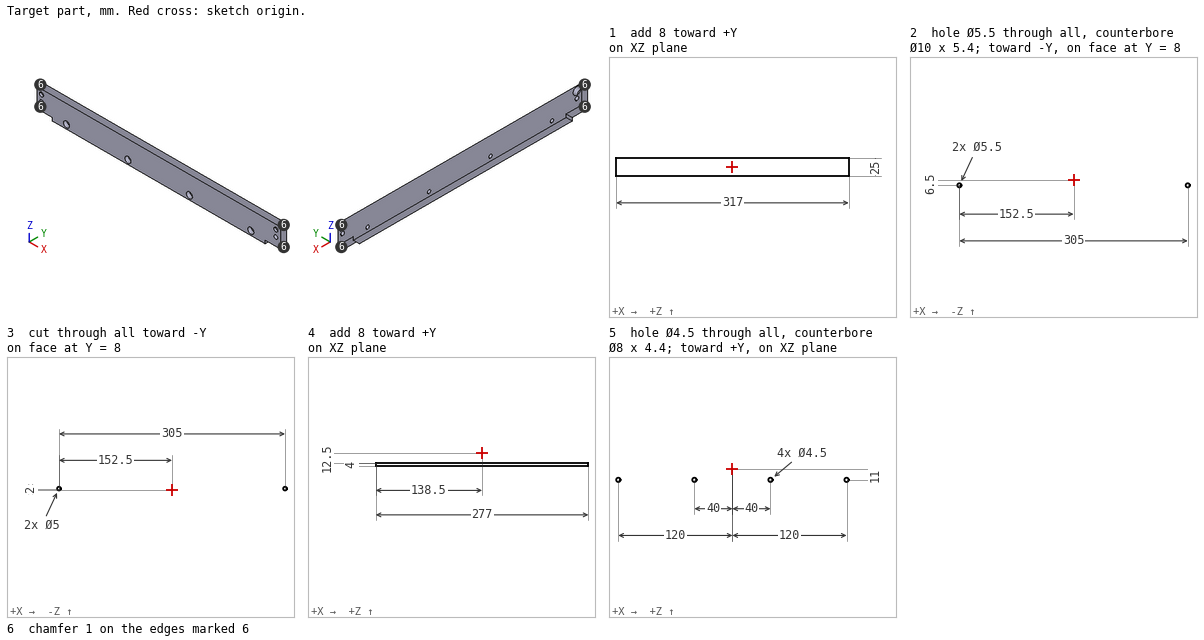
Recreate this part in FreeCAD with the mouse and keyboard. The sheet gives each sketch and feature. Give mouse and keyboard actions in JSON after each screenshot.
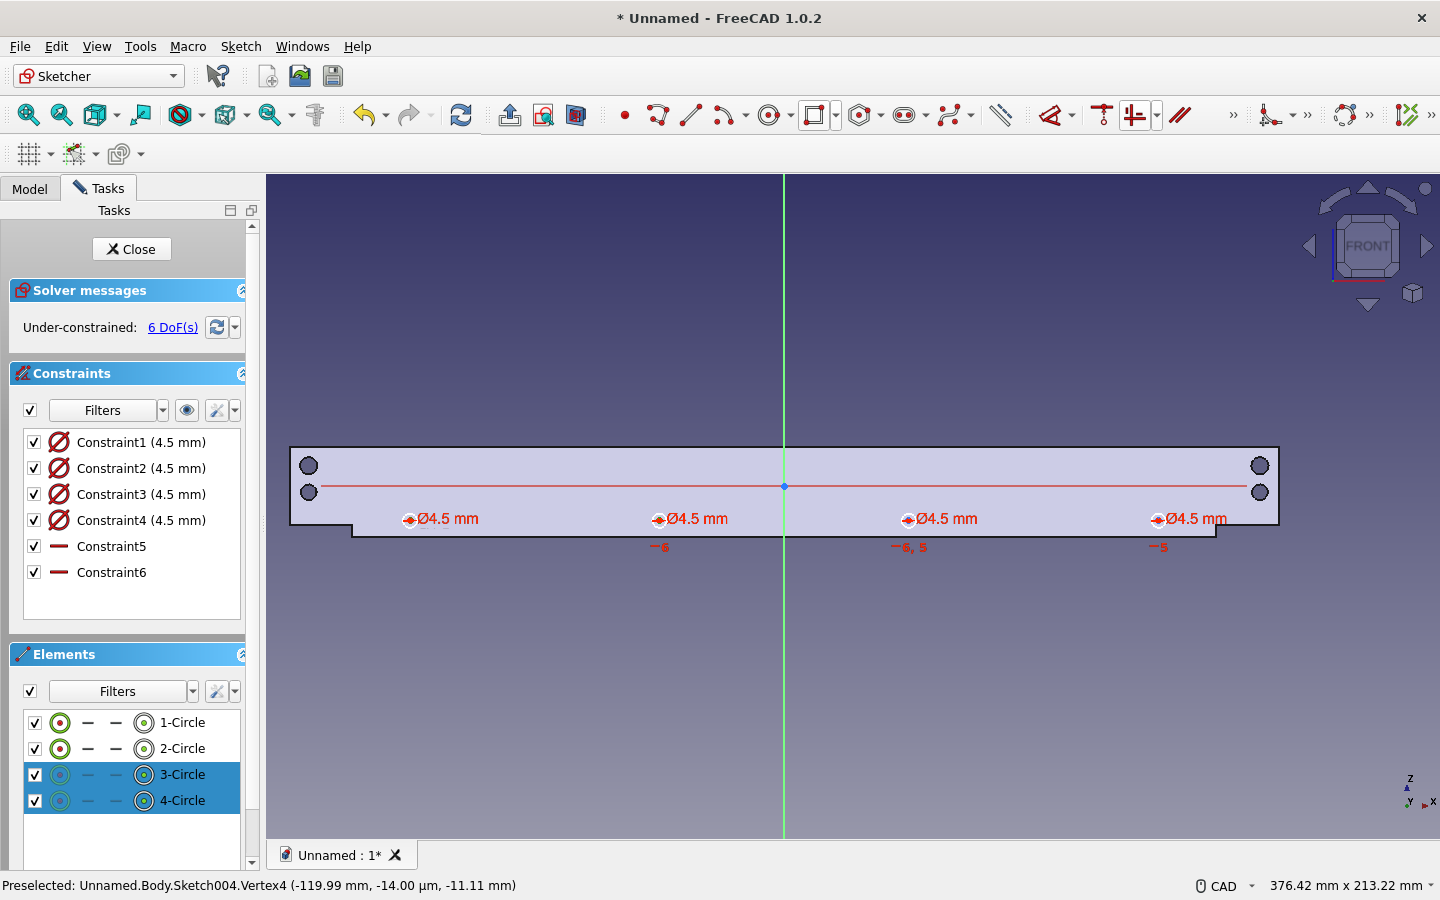
{"action": "left_click", "coordinate": [1156, 116]}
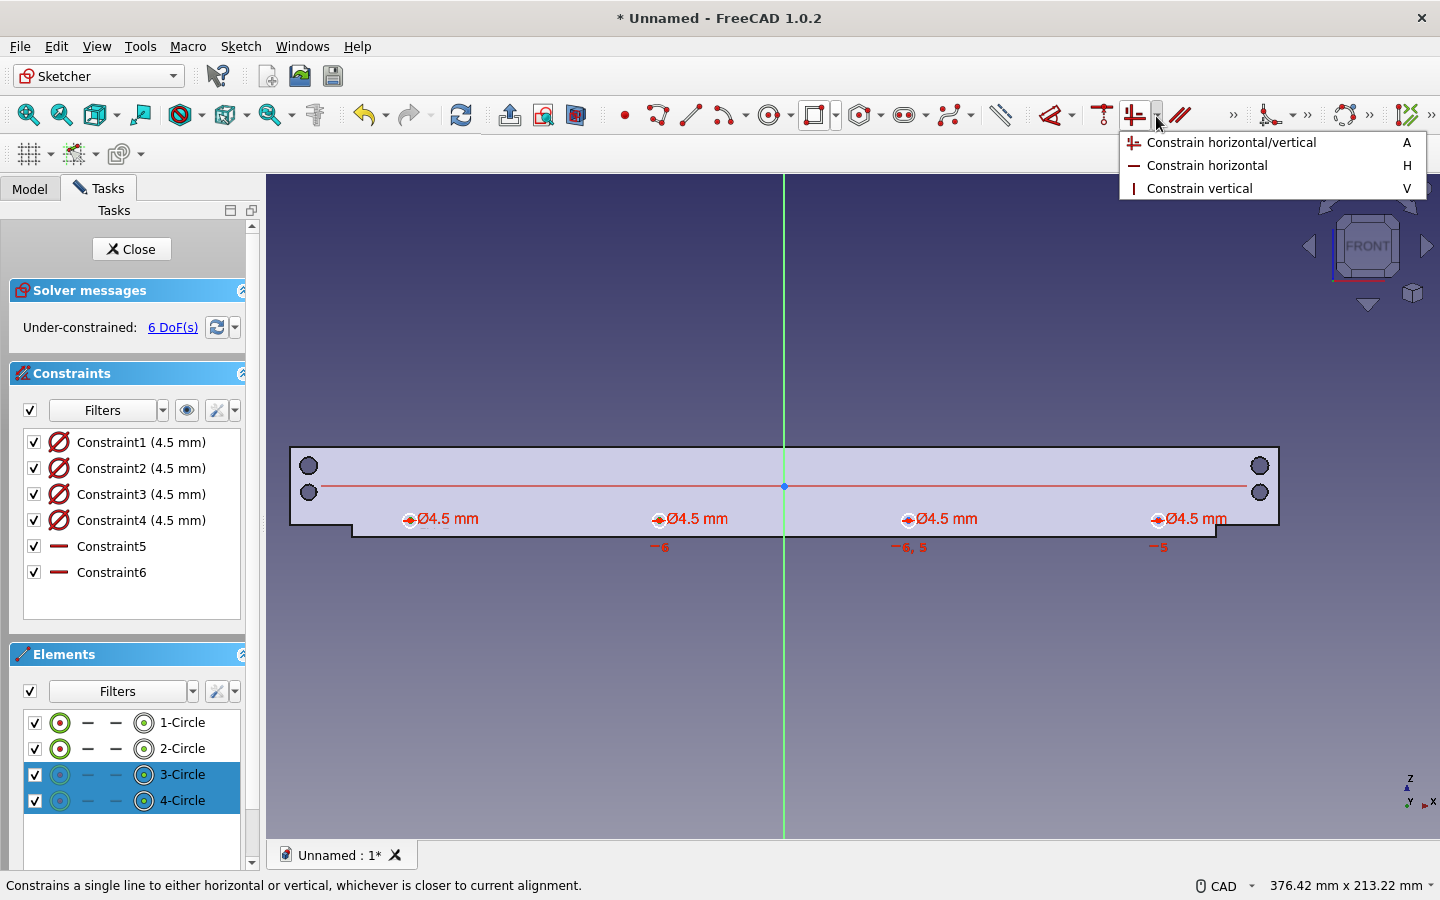
{"action": "left_click", "coordinate": [1273, 166]}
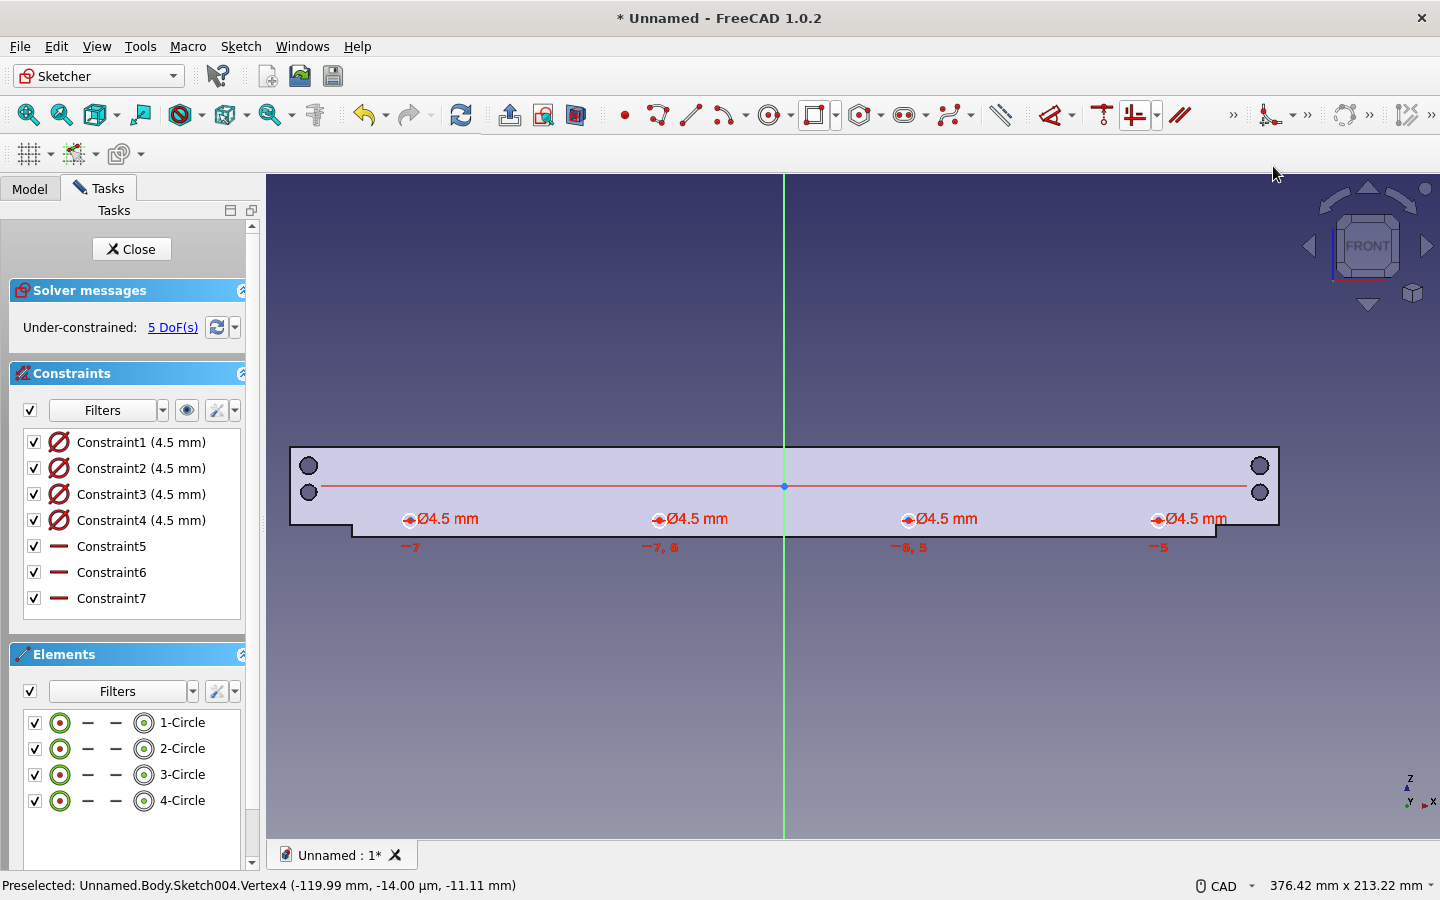
{"action": "left_click", "coordinate": [1050, 116]}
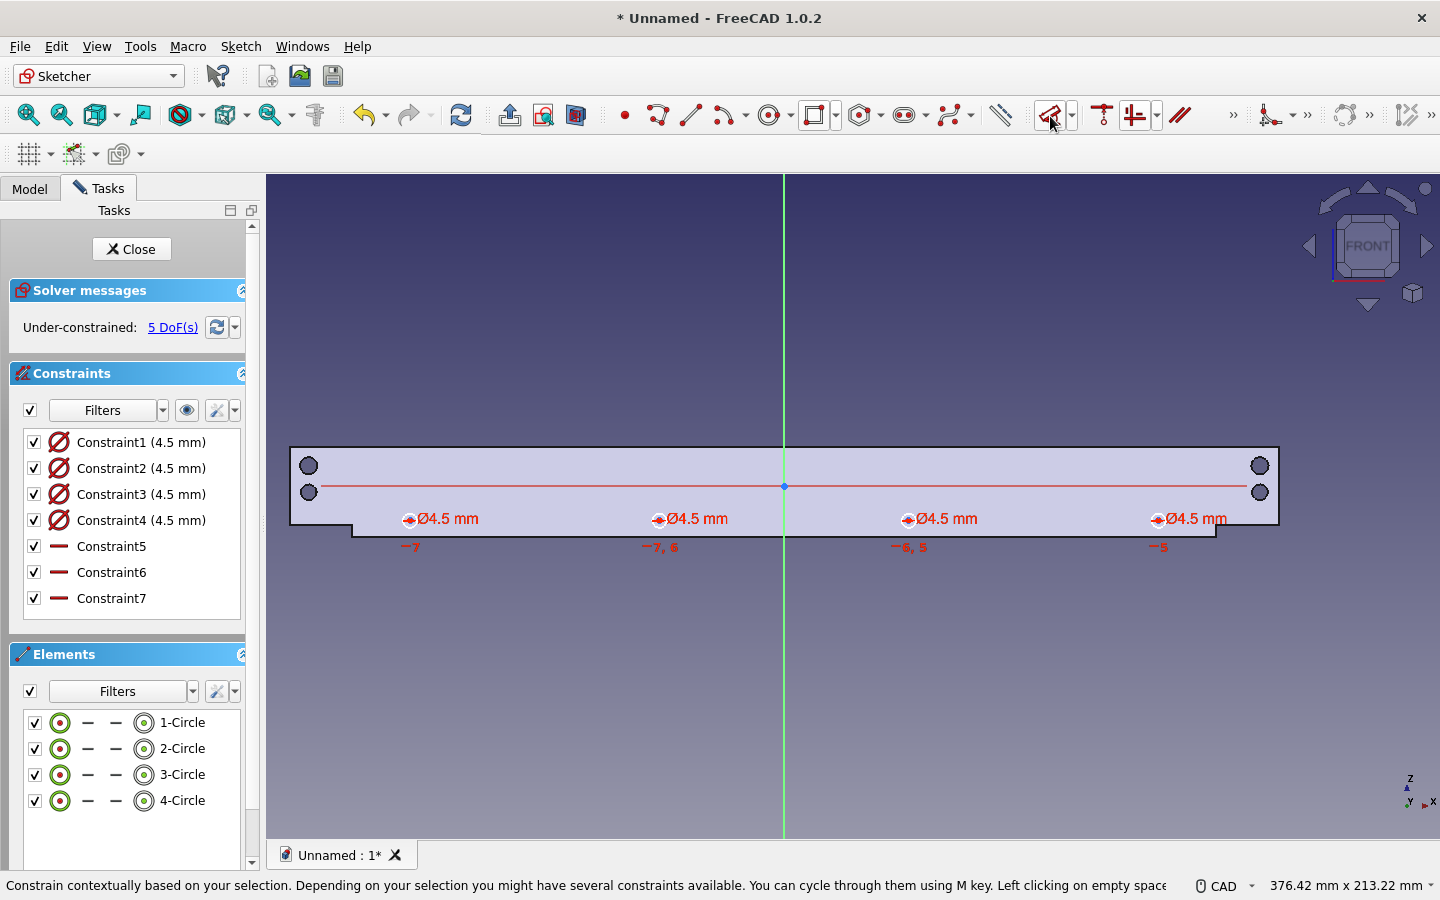
{"action": "left_click", "coordinate": [1159, 521]}
{"action": "left_click", "coordinate": [1193, 503]}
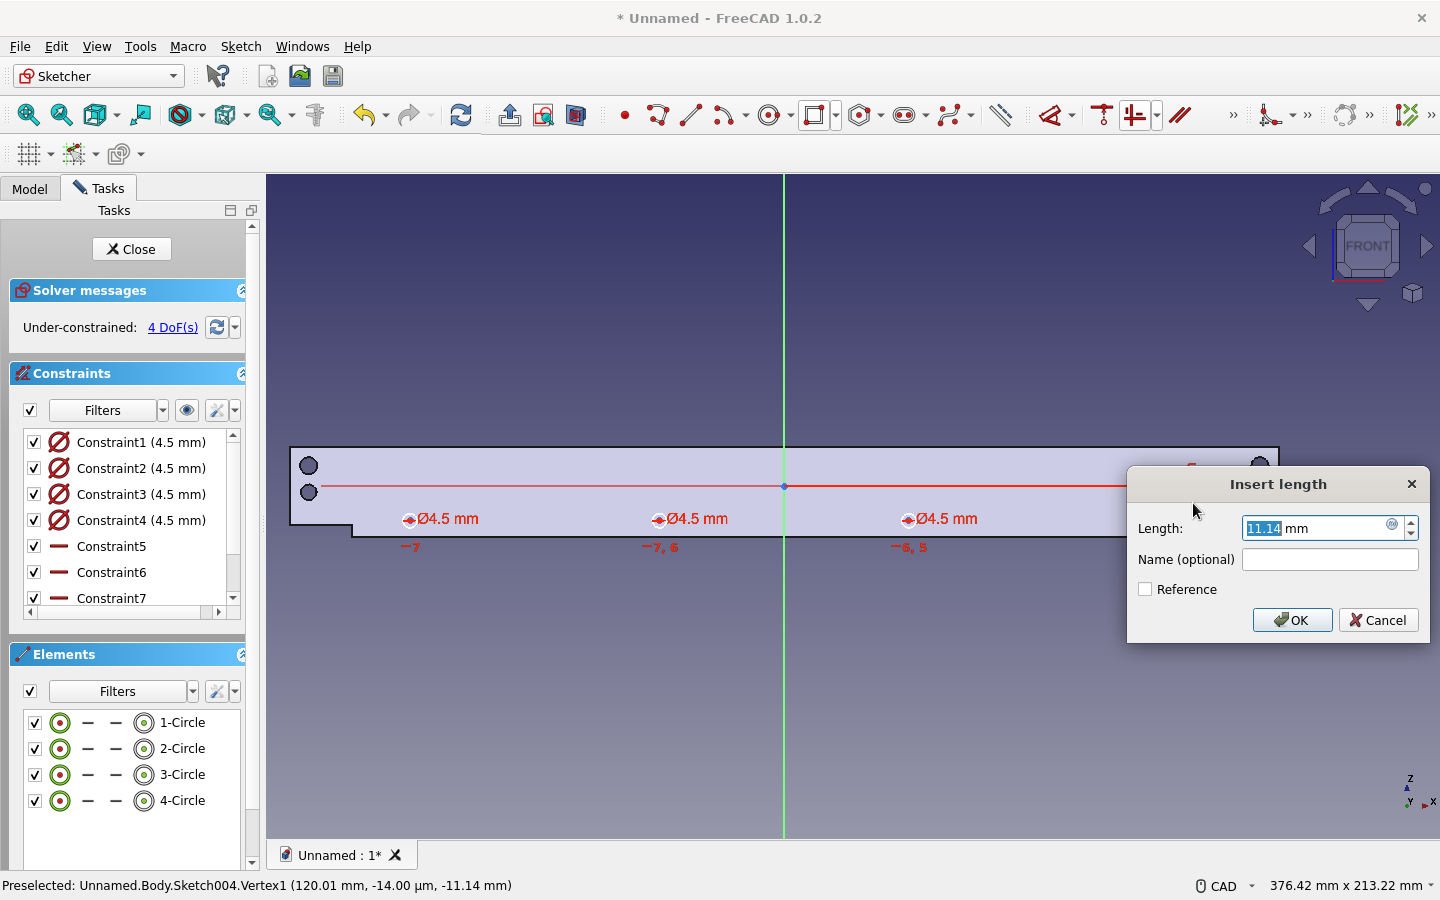
{"action": "type", "text": "11"}
{"action": "key", "text": "Return"}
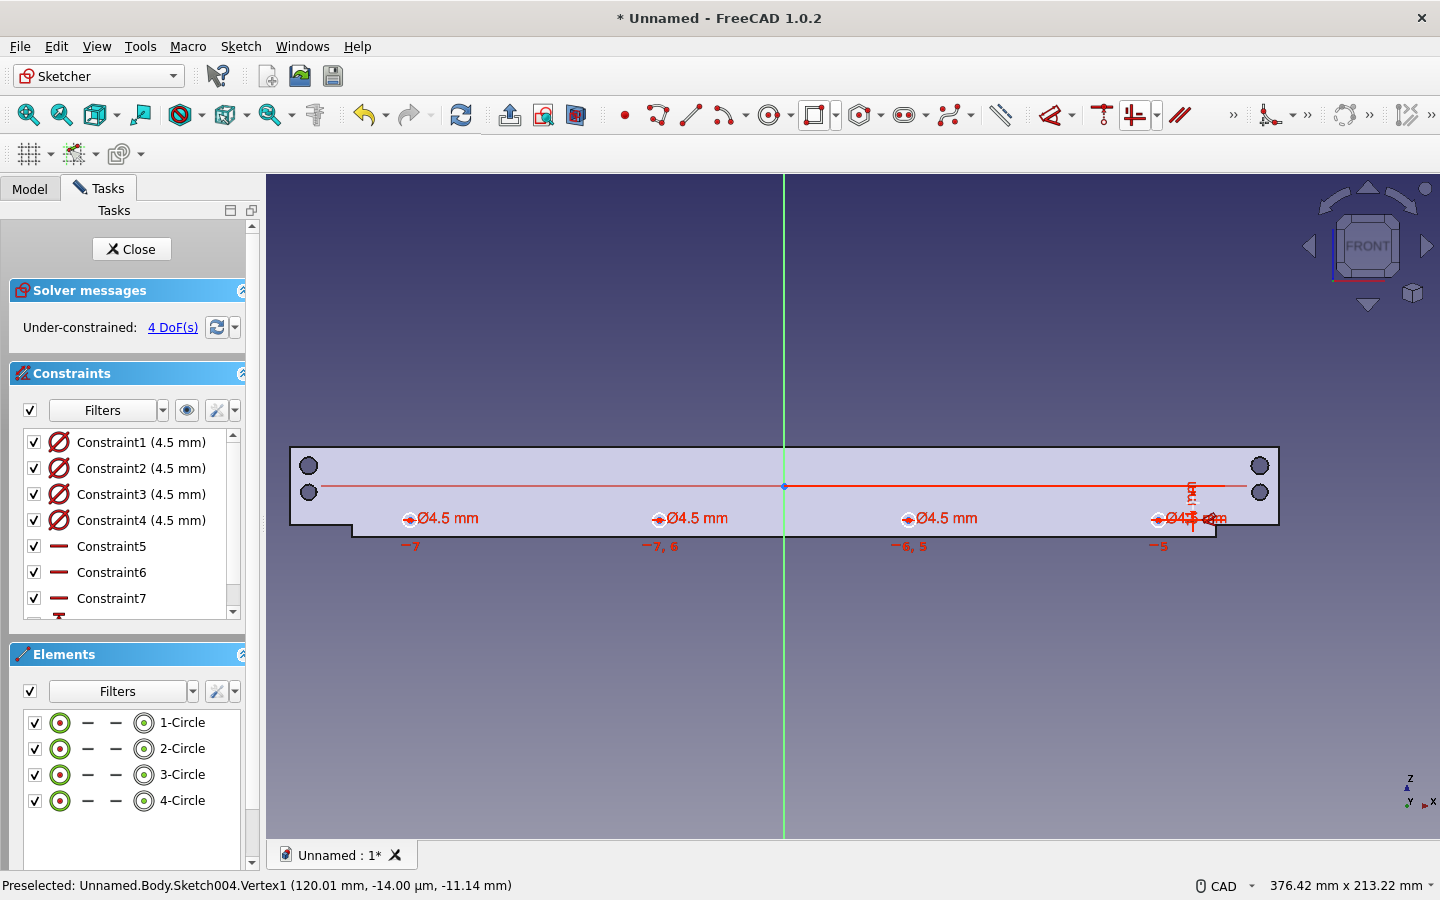
{"action": "left_click", "coordinate": [909, 520]}
{"action": "left_click", "coordinate": [847, 452]}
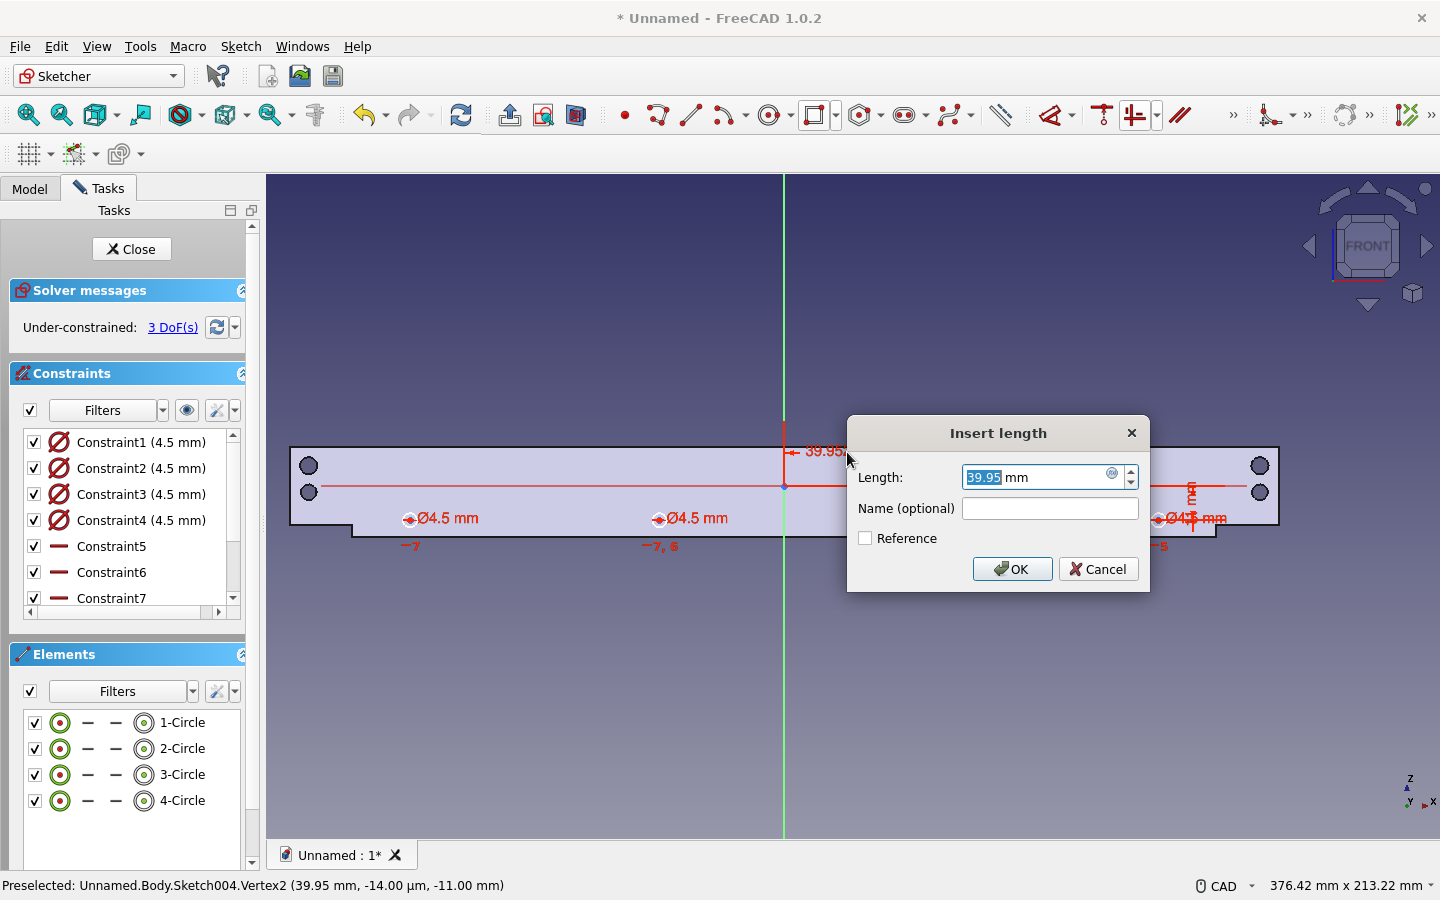
{"action": "type", "text": "40"}
{"action": "key", "text": "Return"}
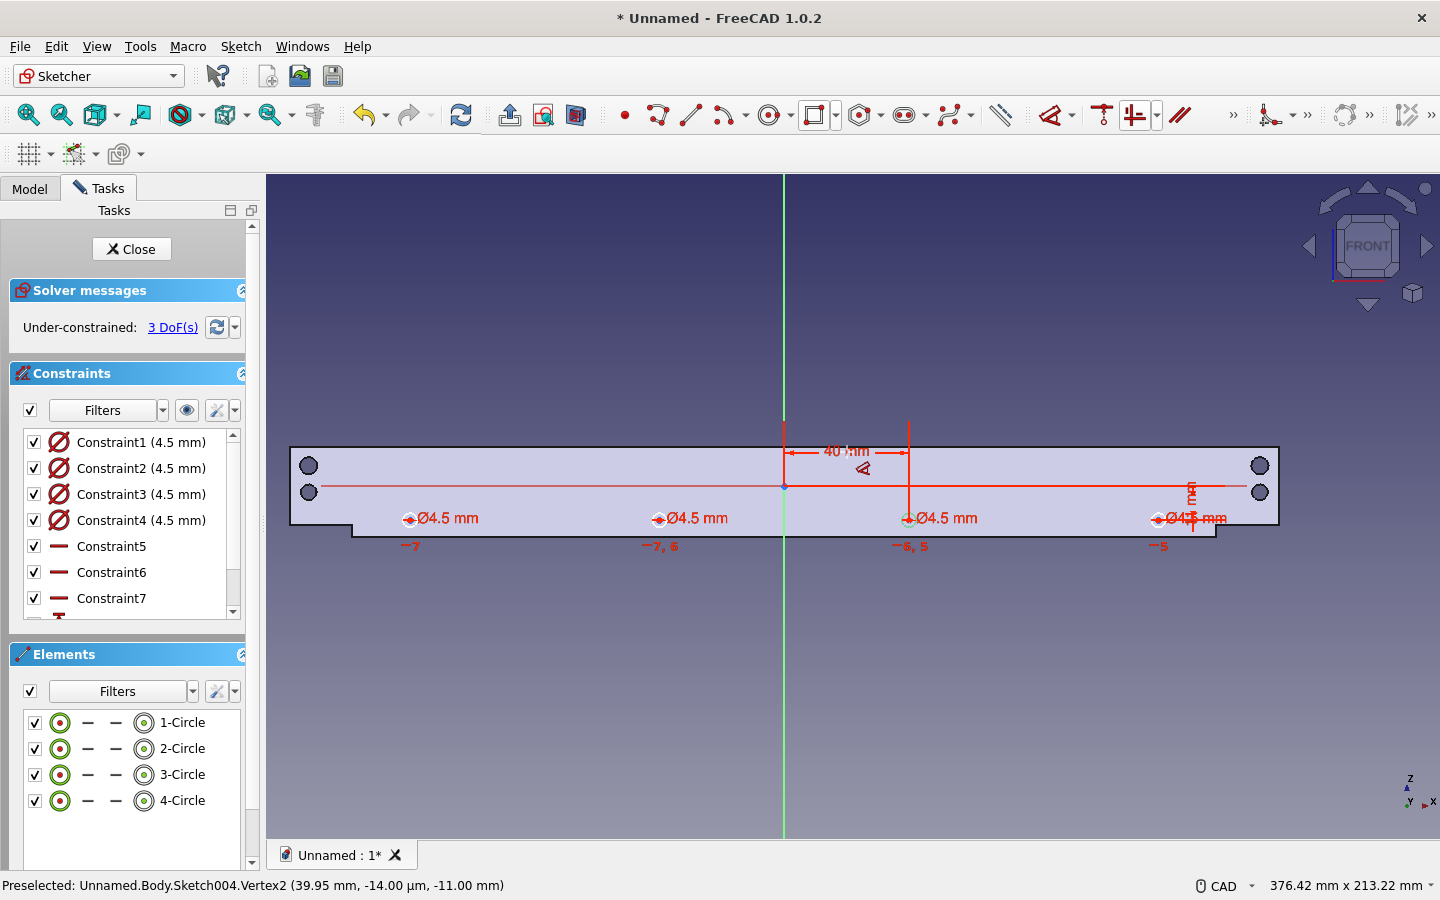
{"action": "left_click", "coordinate": [660, 520]}
{"action": "left_click", "coordinate": [722, 452]}